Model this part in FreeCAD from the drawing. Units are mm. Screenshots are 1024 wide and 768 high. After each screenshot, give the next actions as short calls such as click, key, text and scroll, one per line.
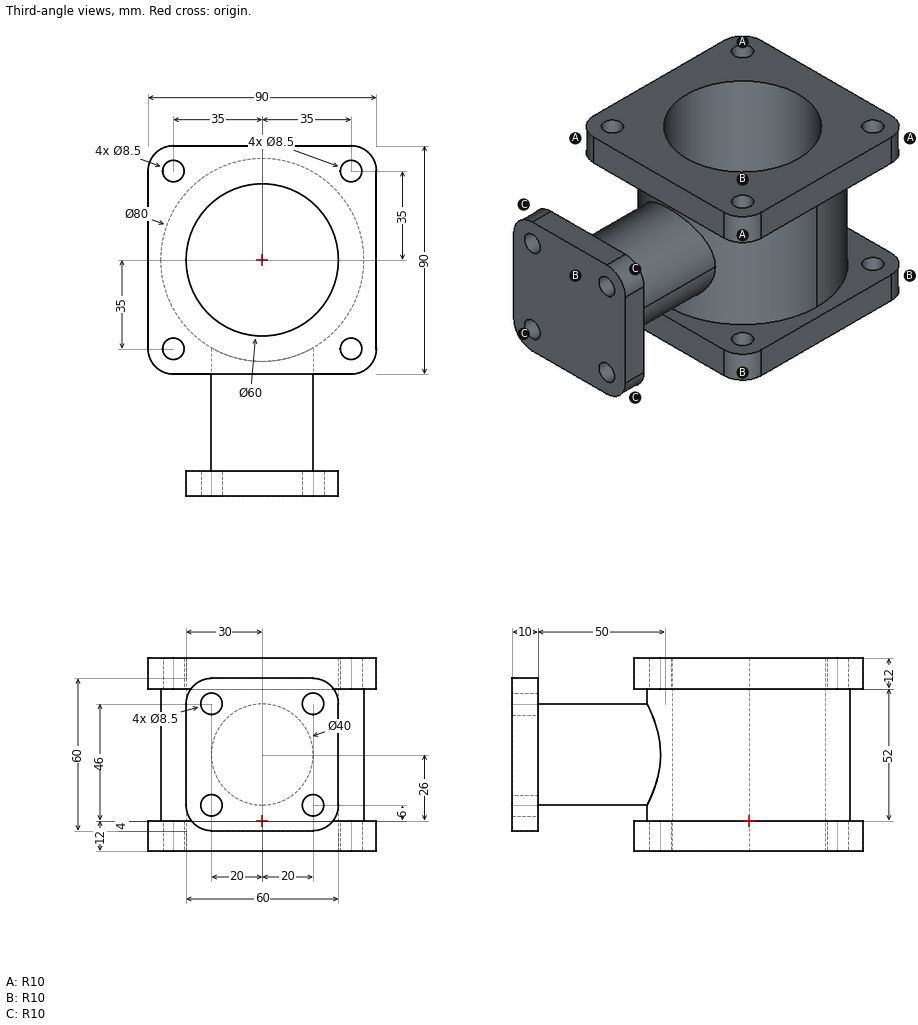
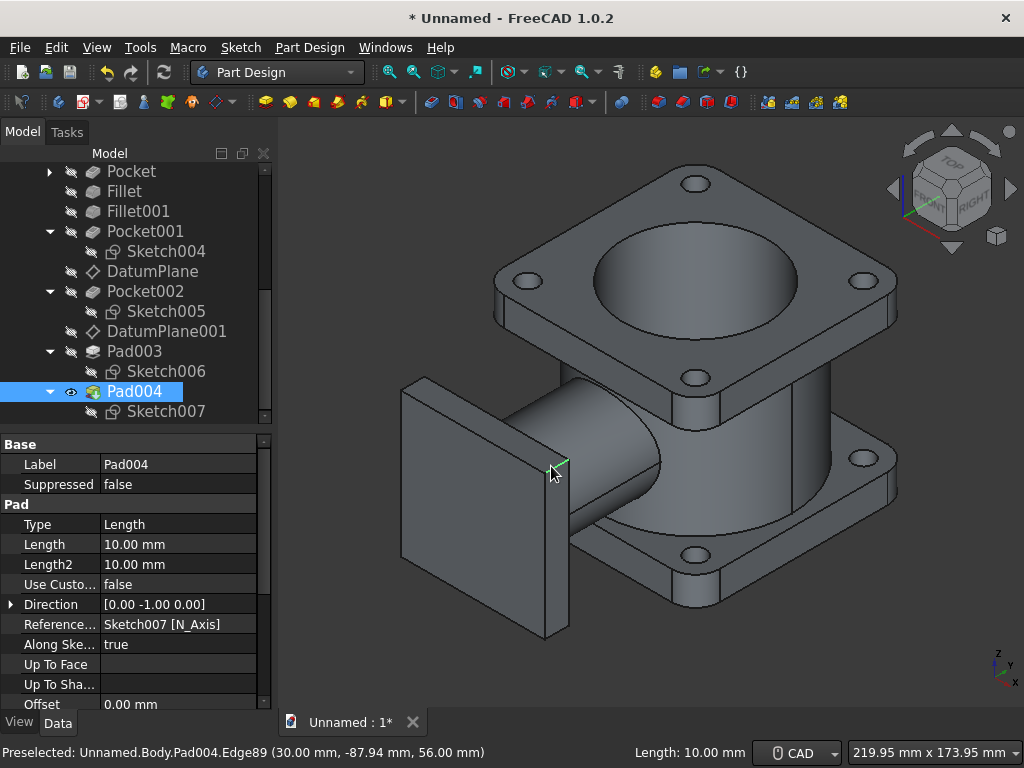
key(2)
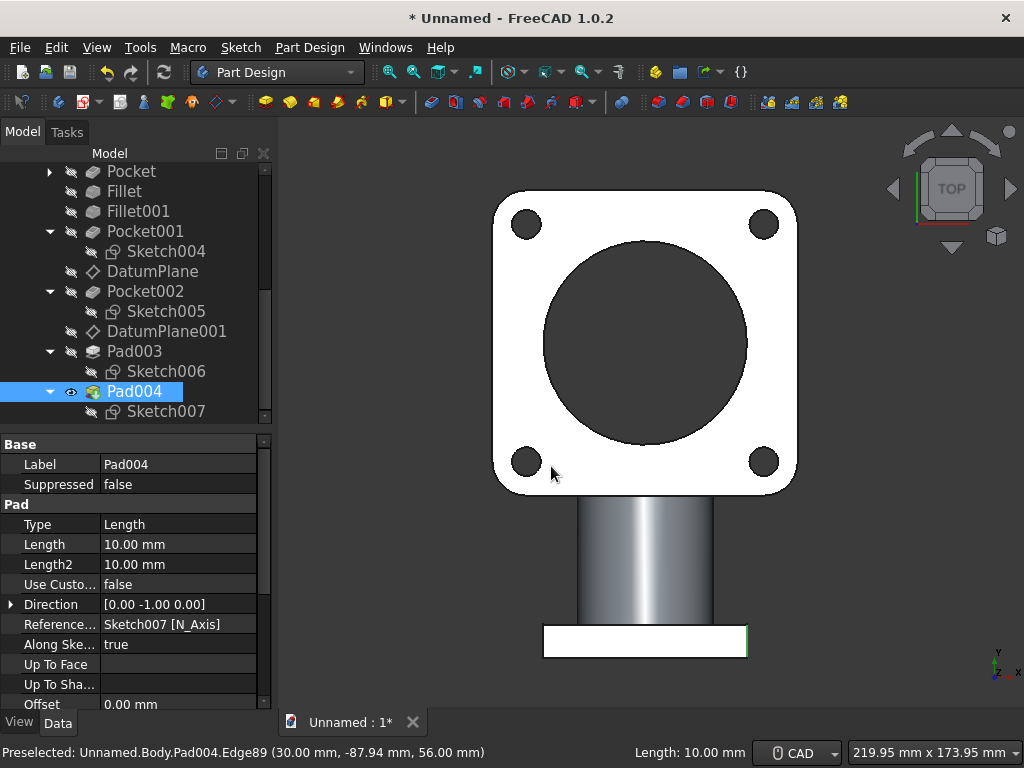
click(543, 640, ctrl)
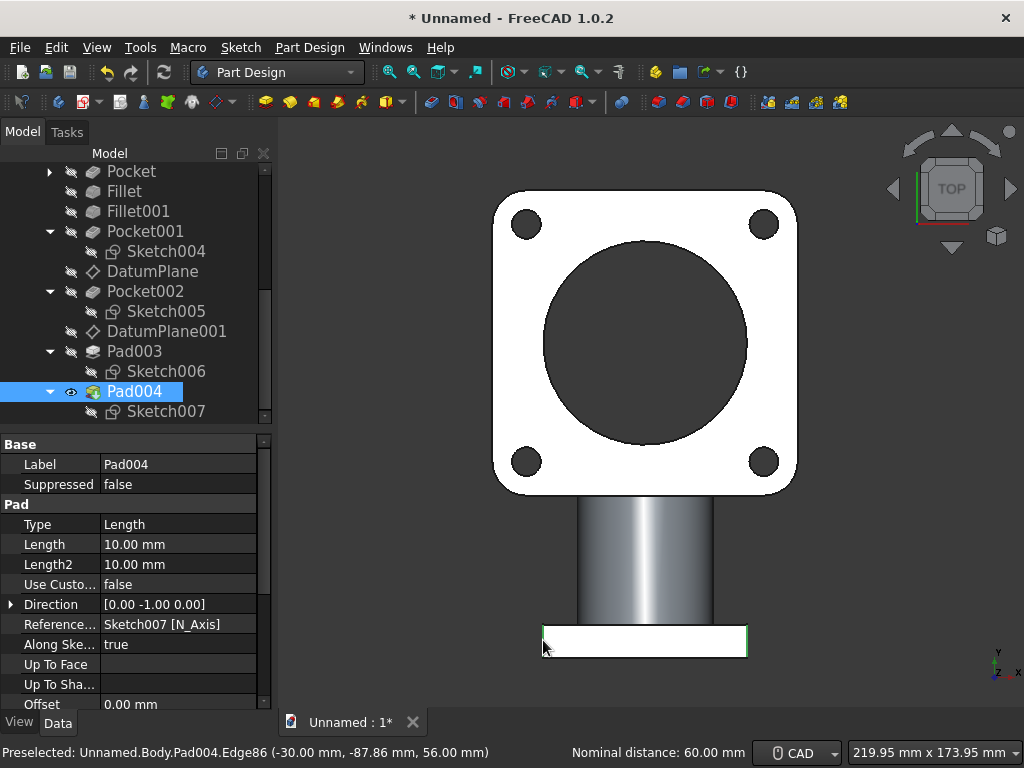
key(0)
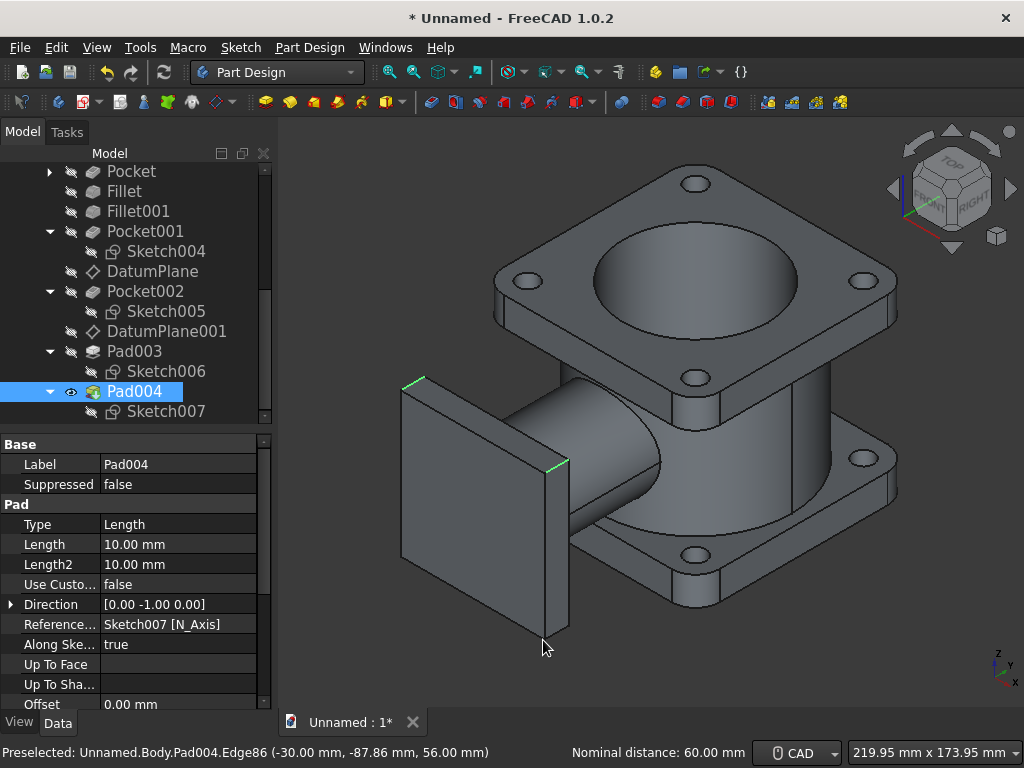
key(1)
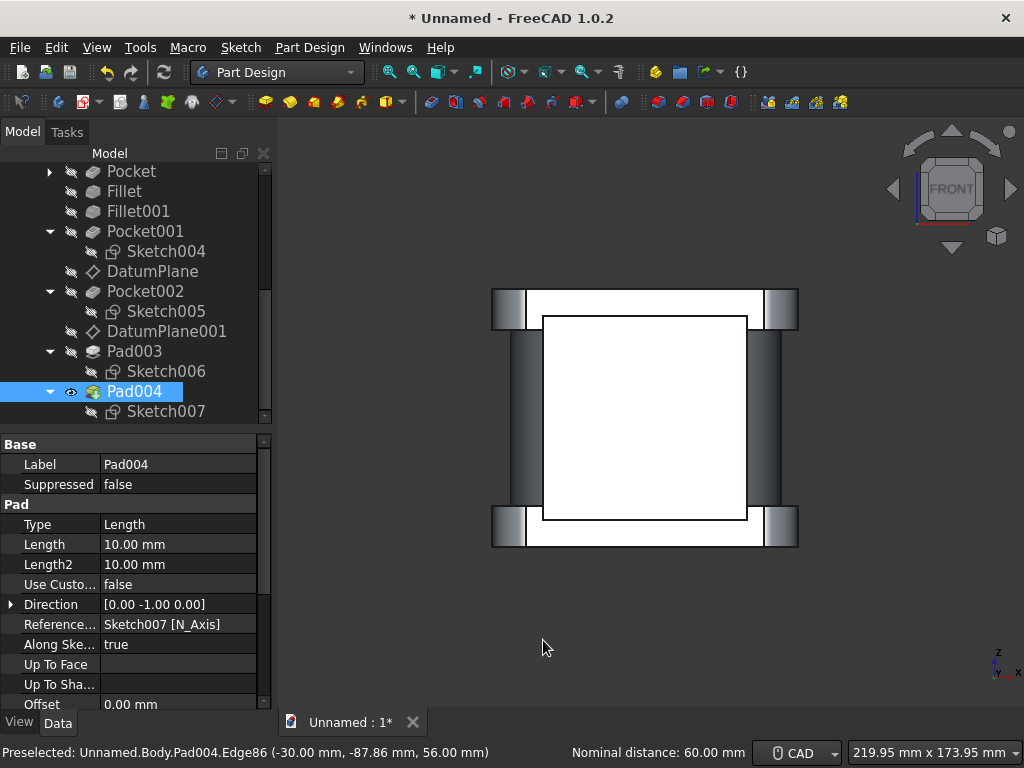
click(390, 72)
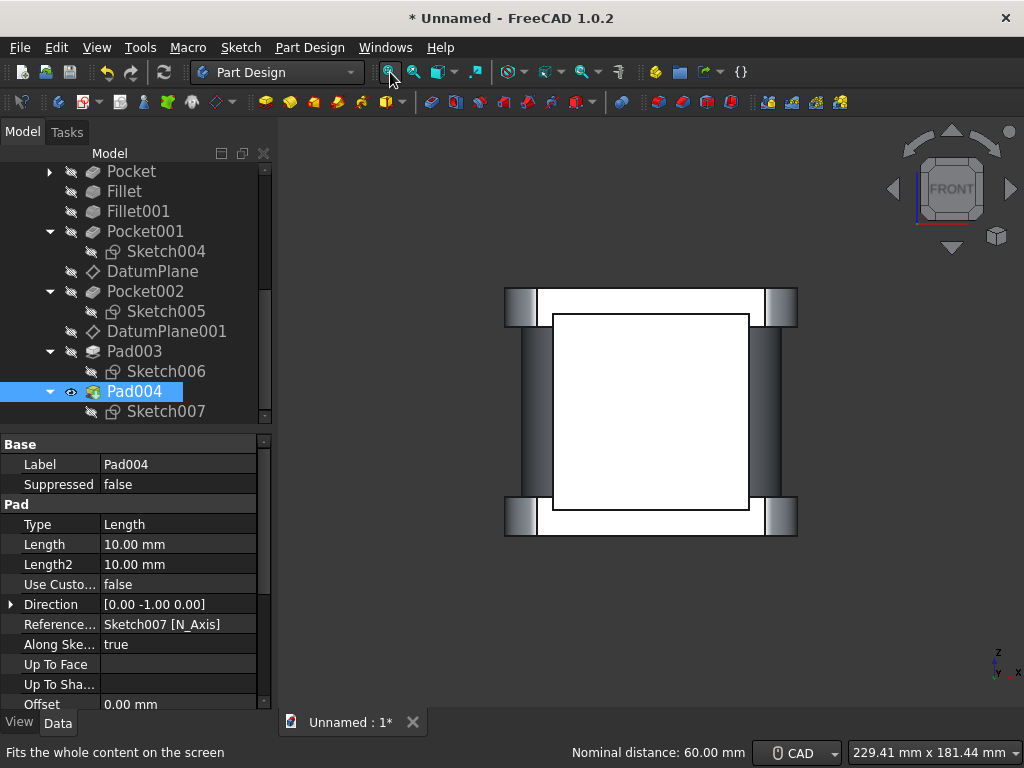
key(3)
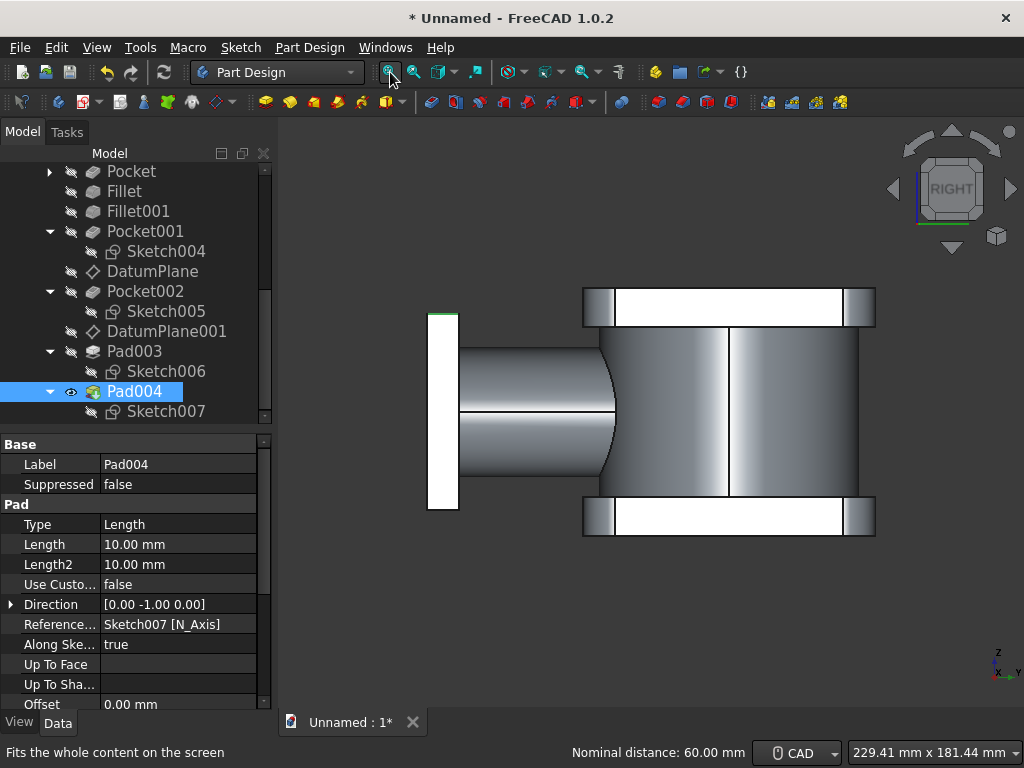
click(443, 509, ctrl)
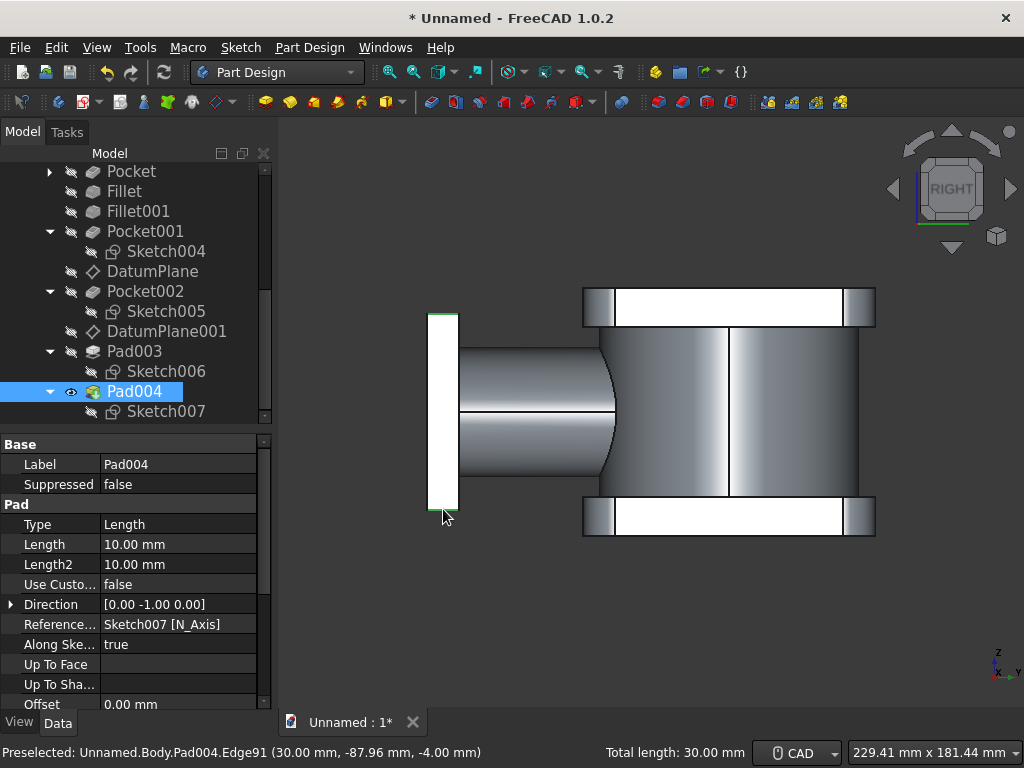
key(5)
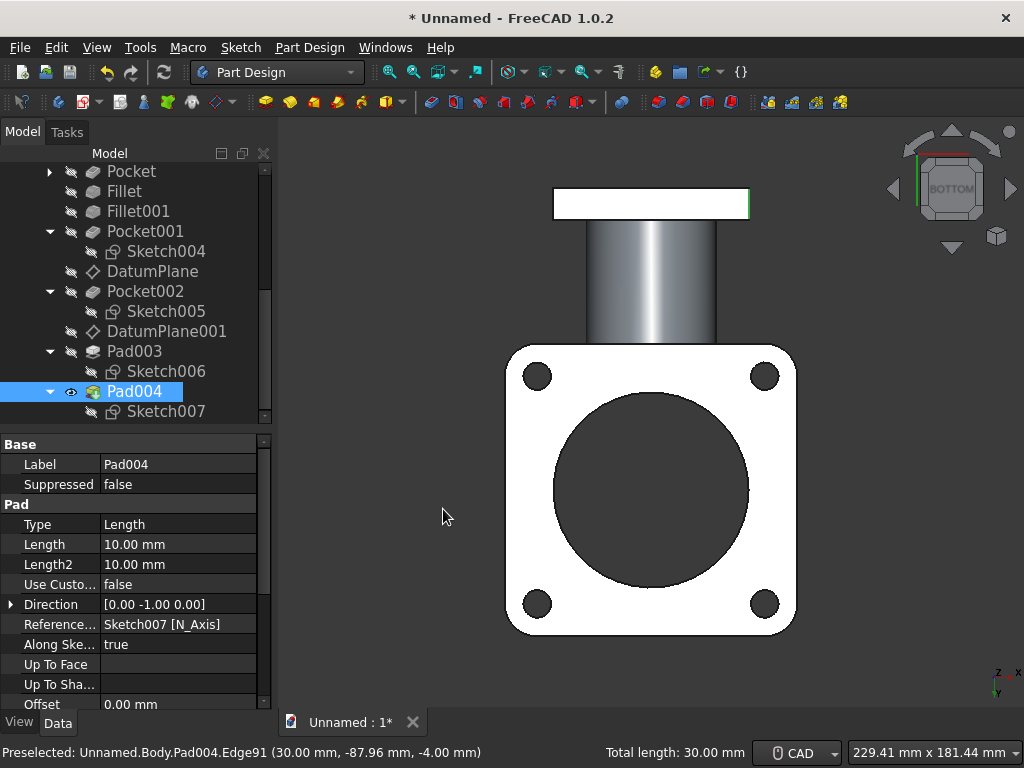
click(553, 203, ctrl)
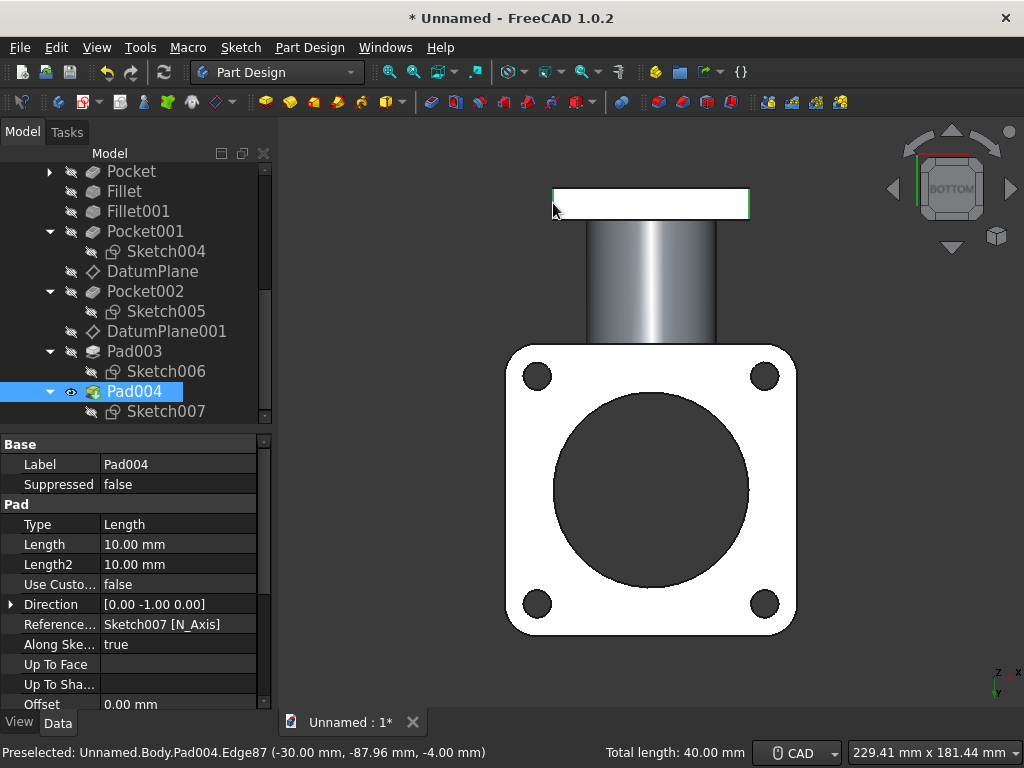
click(660, 102)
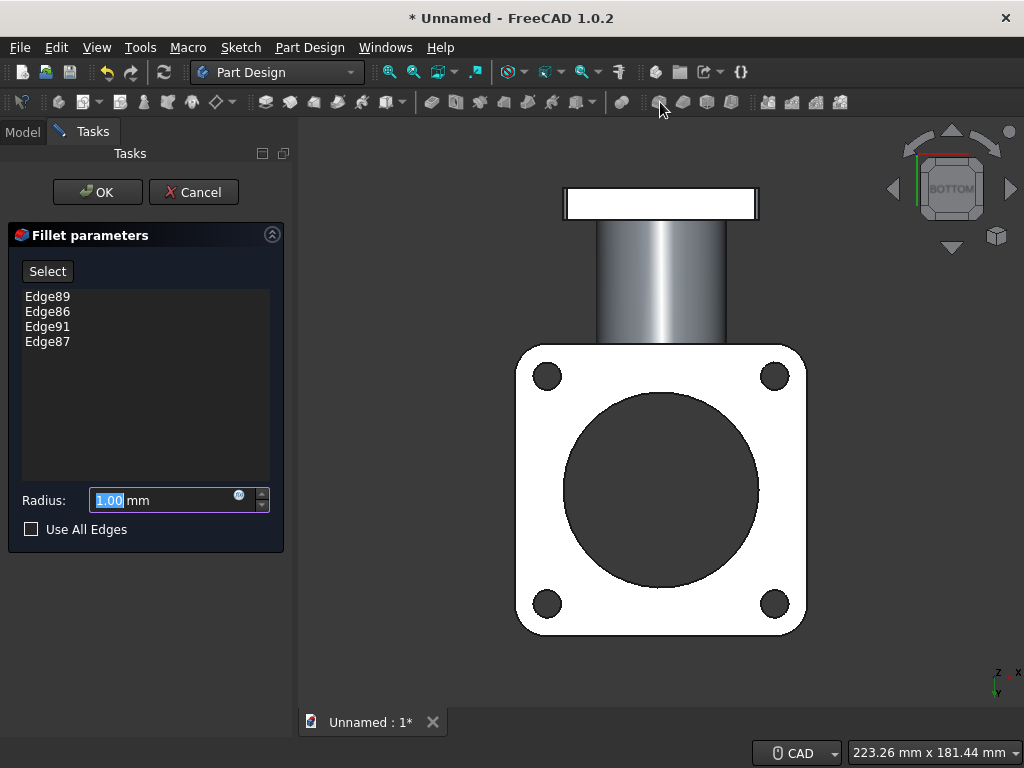
text(10)
key(Tab)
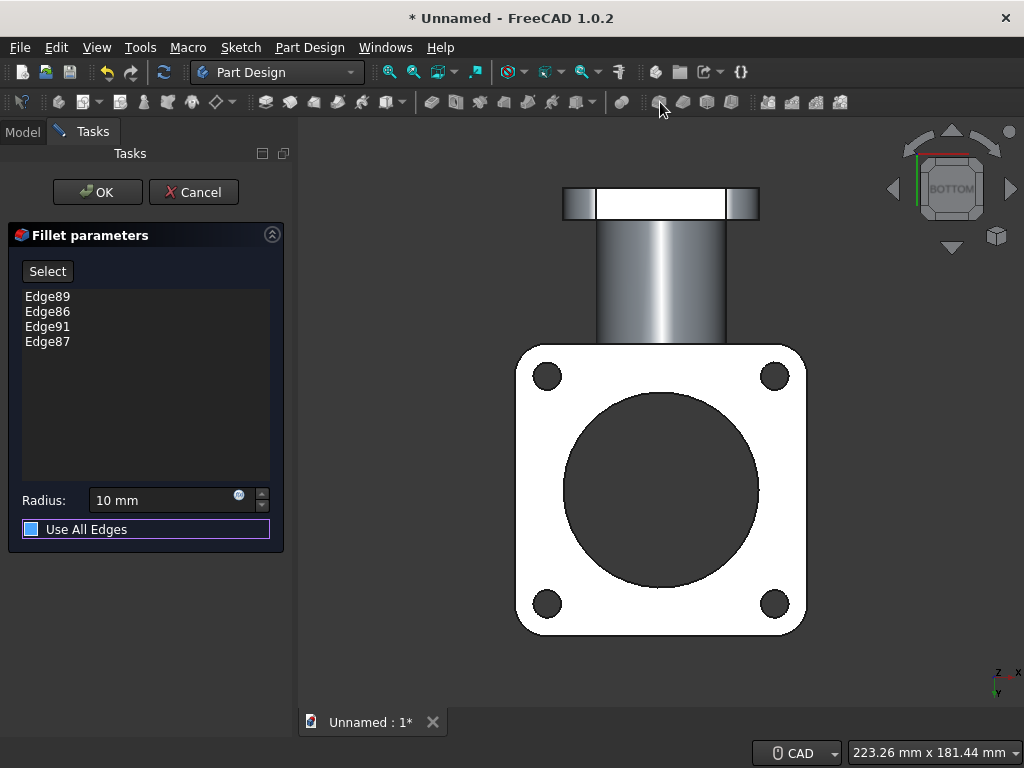
click(98, 192)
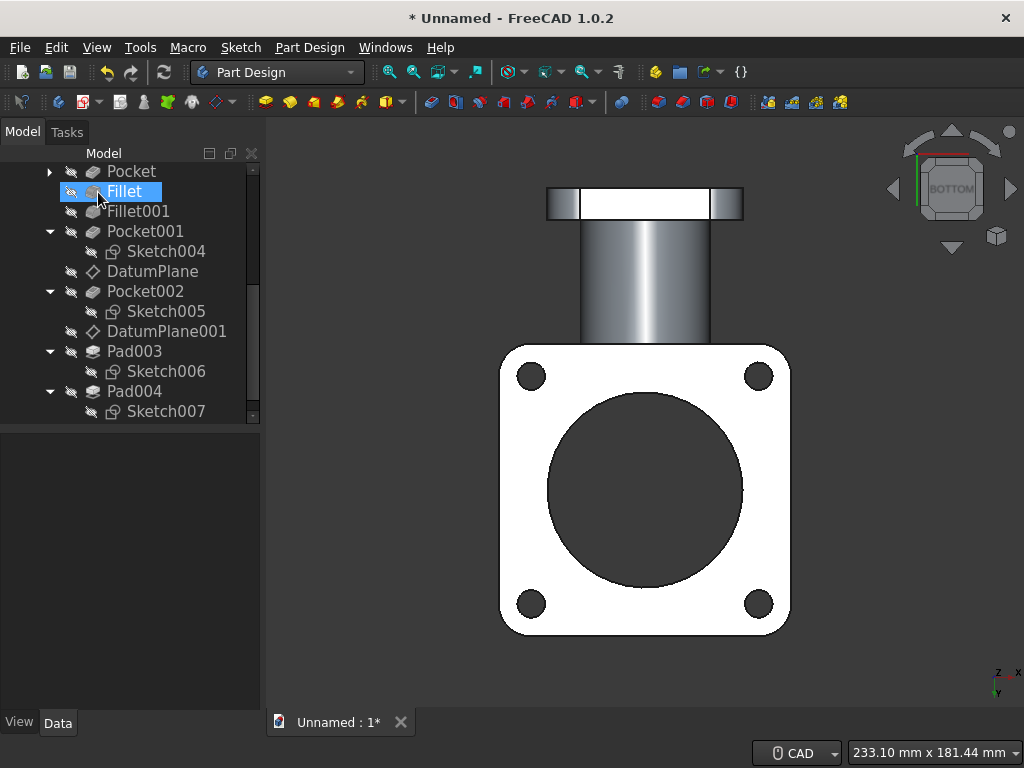
key(0)